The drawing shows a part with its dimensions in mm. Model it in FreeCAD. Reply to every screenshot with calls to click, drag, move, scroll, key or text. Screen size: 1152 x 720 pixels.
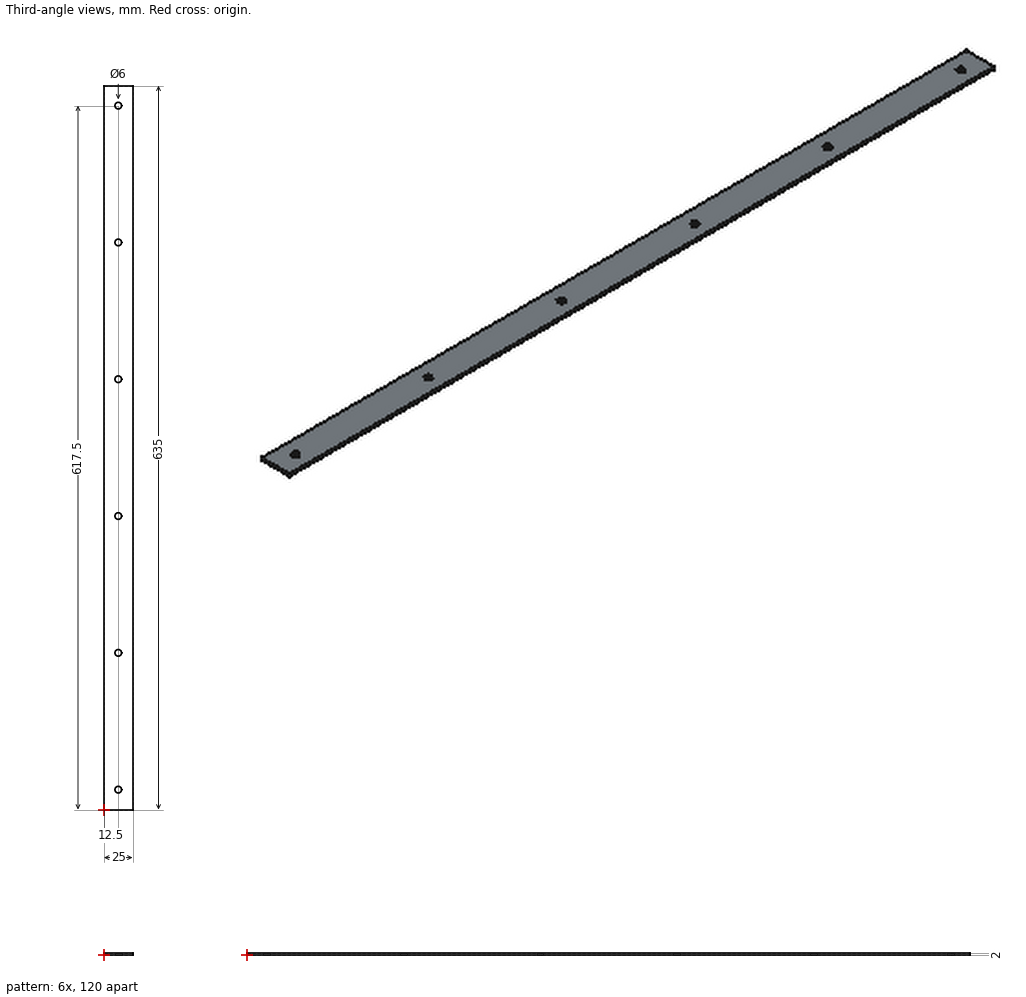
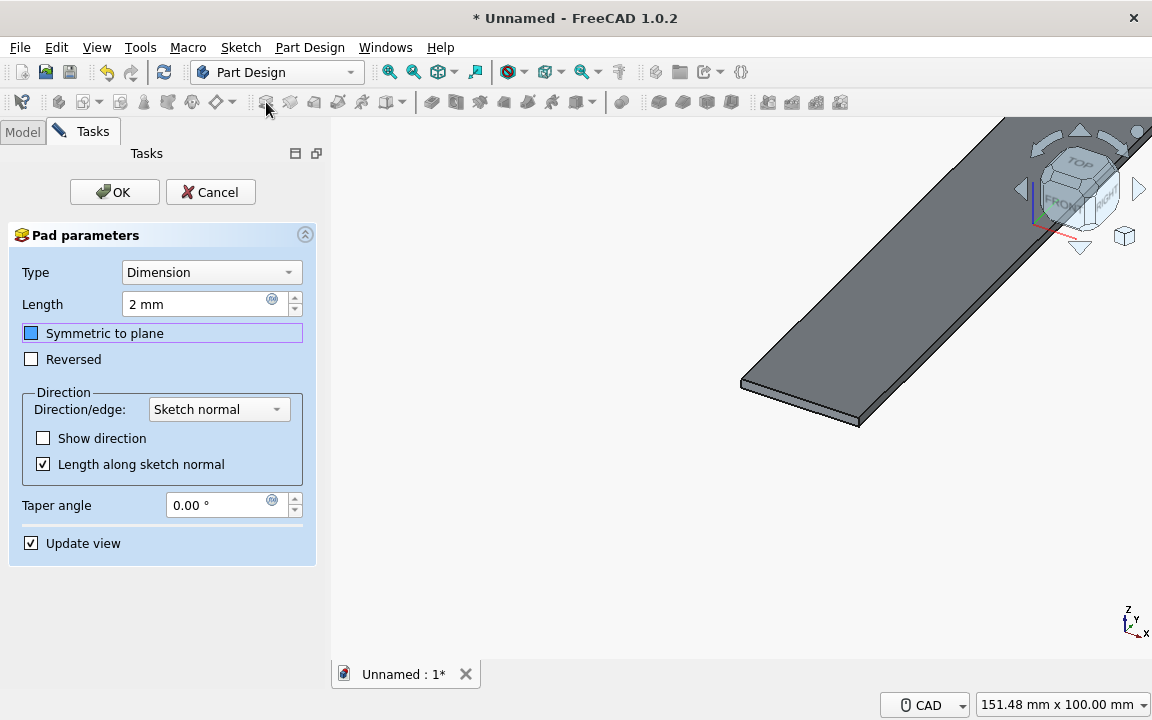
click(115, 192)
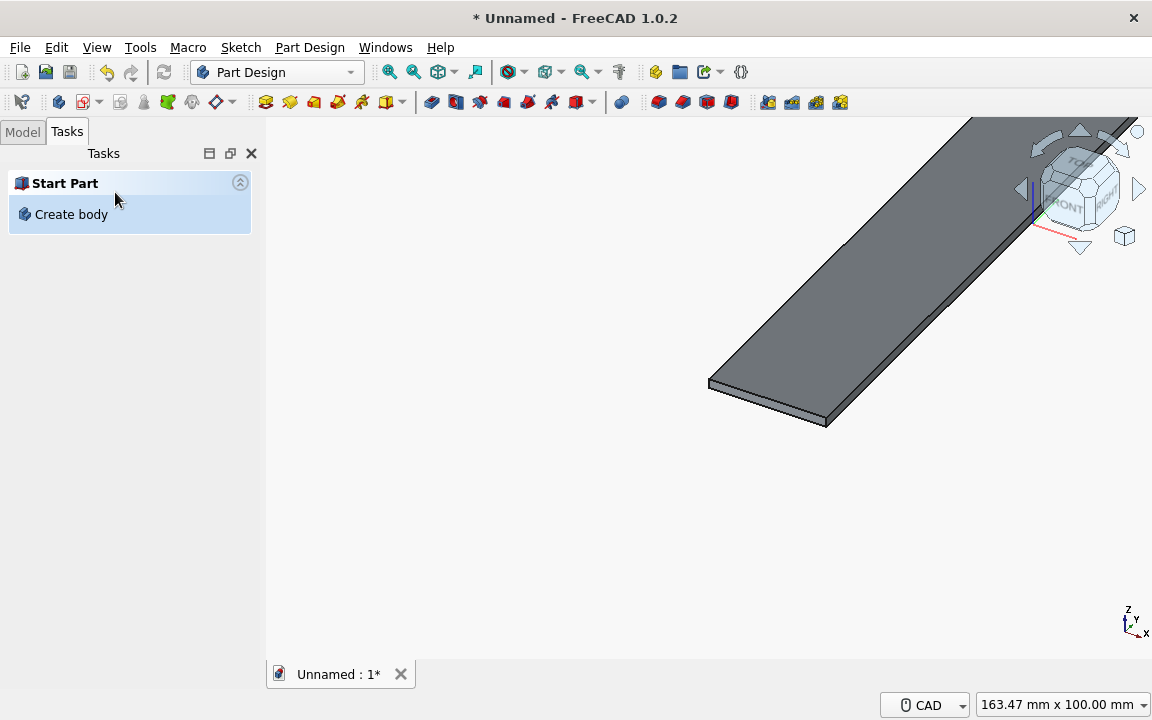
click(390, 72)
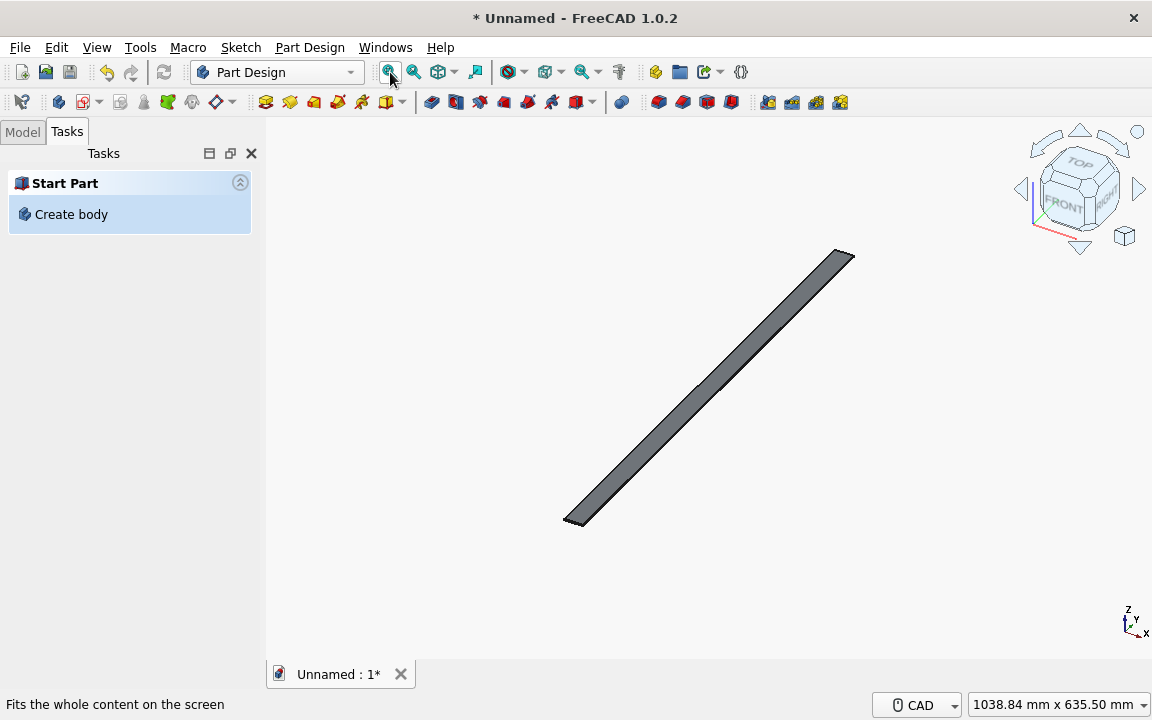
click(786, 309)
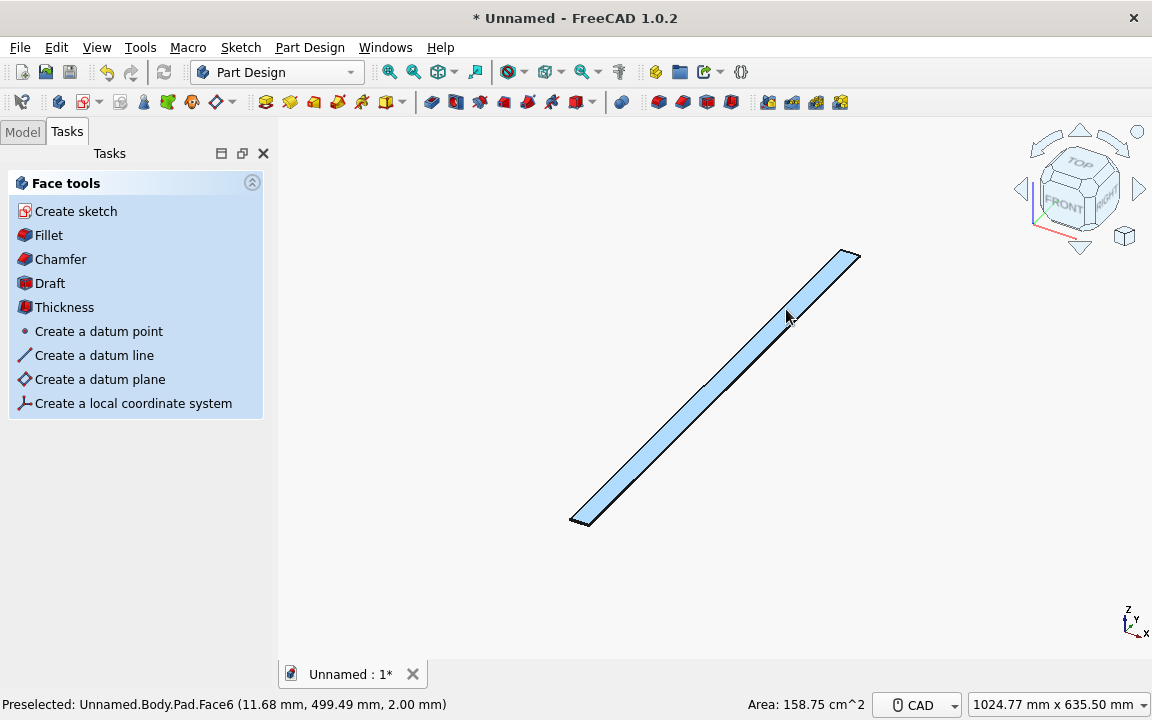
click(84, 102)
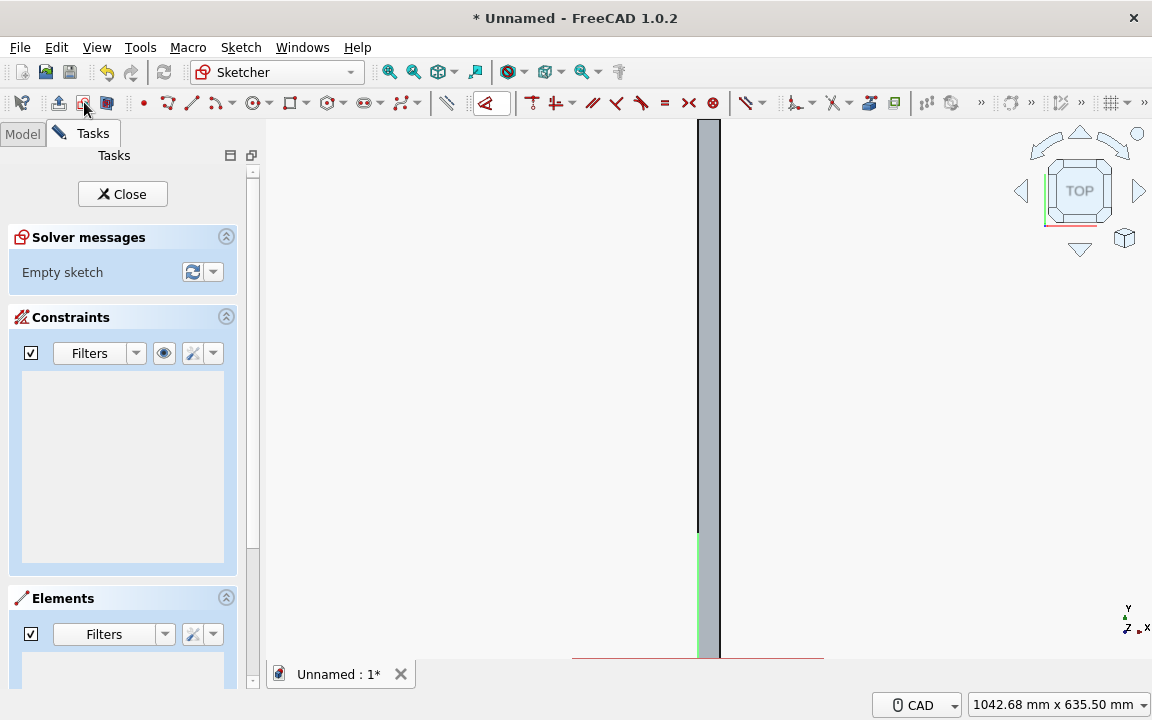
scroll(640, 389, down, 5)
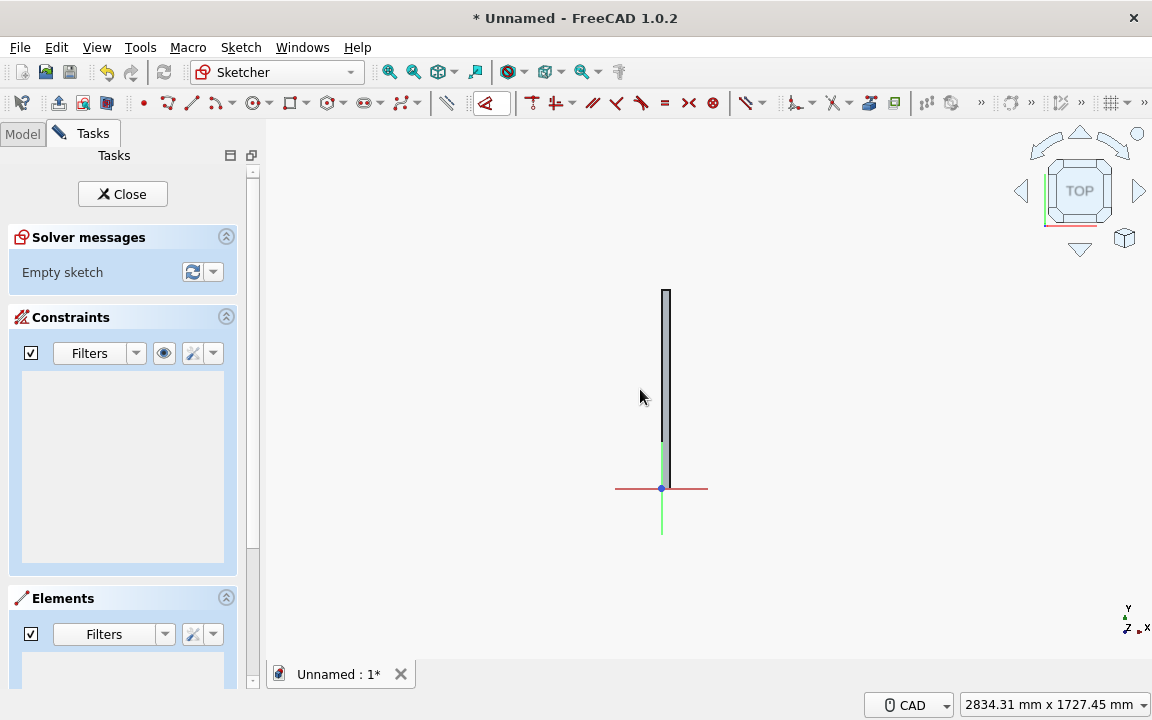
scroll(667, 291, up, 15)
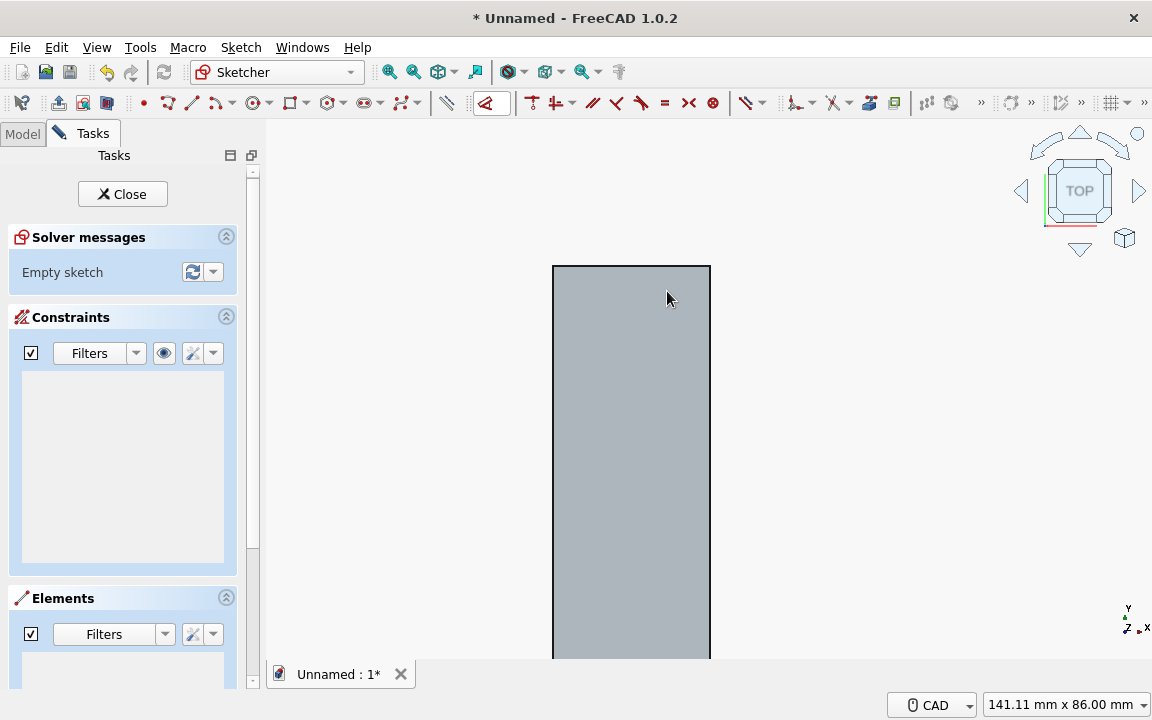
scroll(630, 374, up, 11)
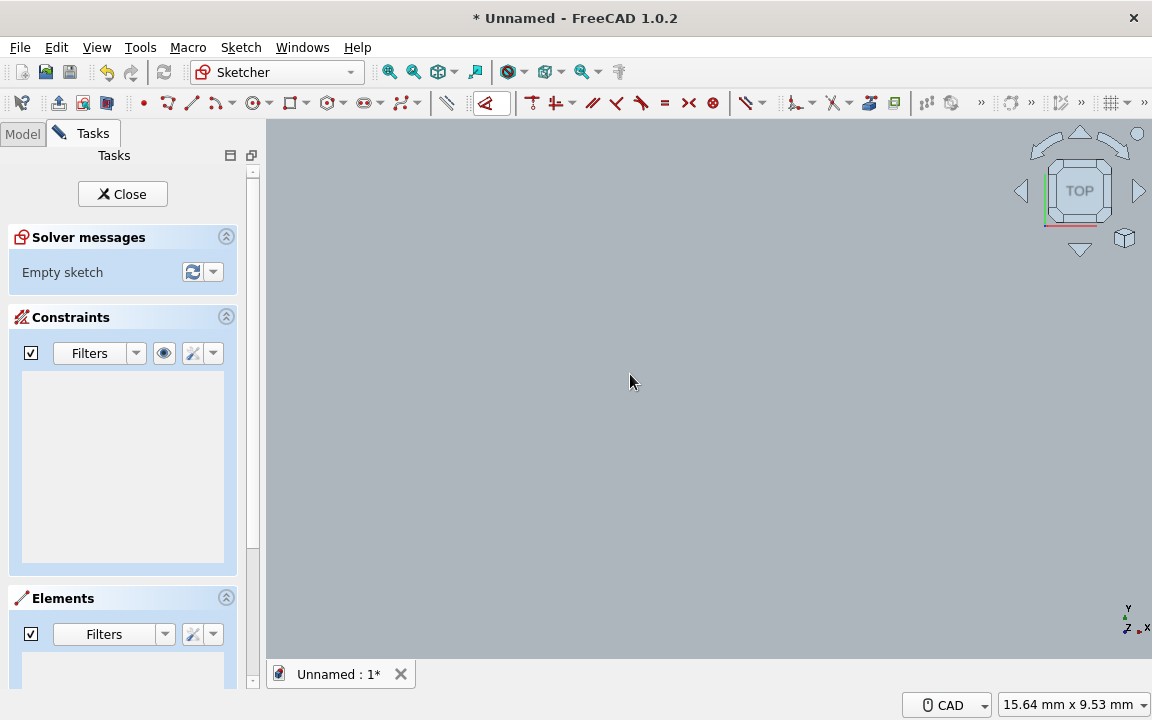
click(254, 104)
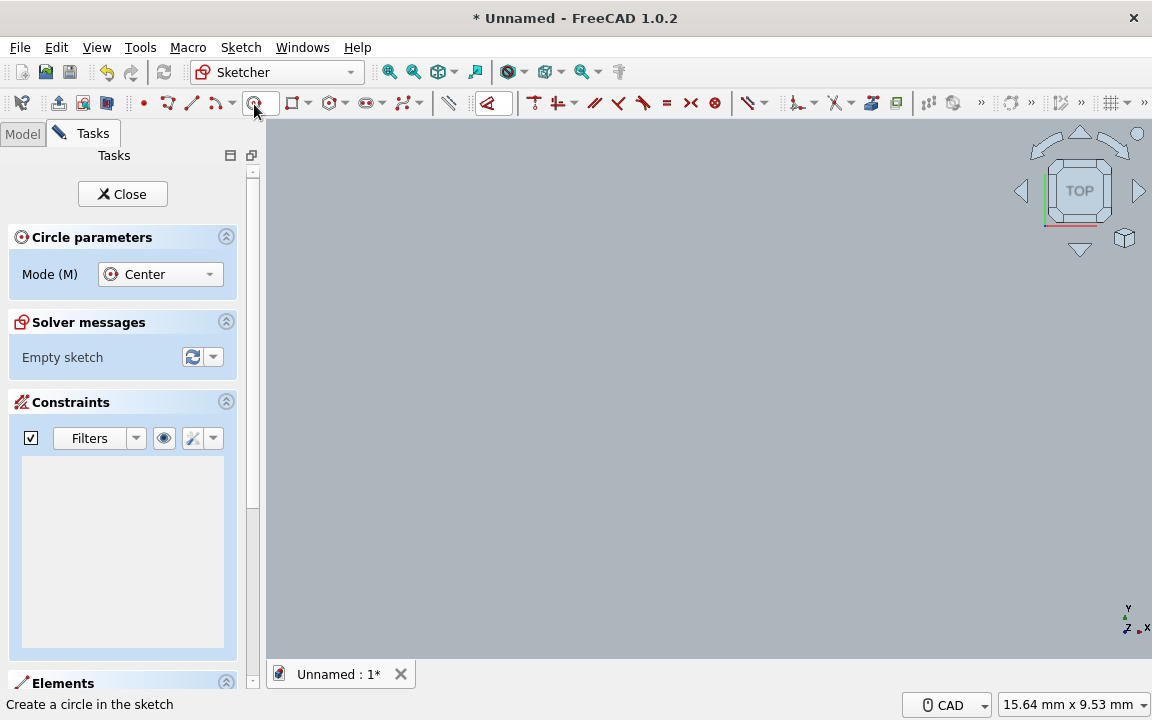
click(638, 389)
click(758, 268)
key(Escape)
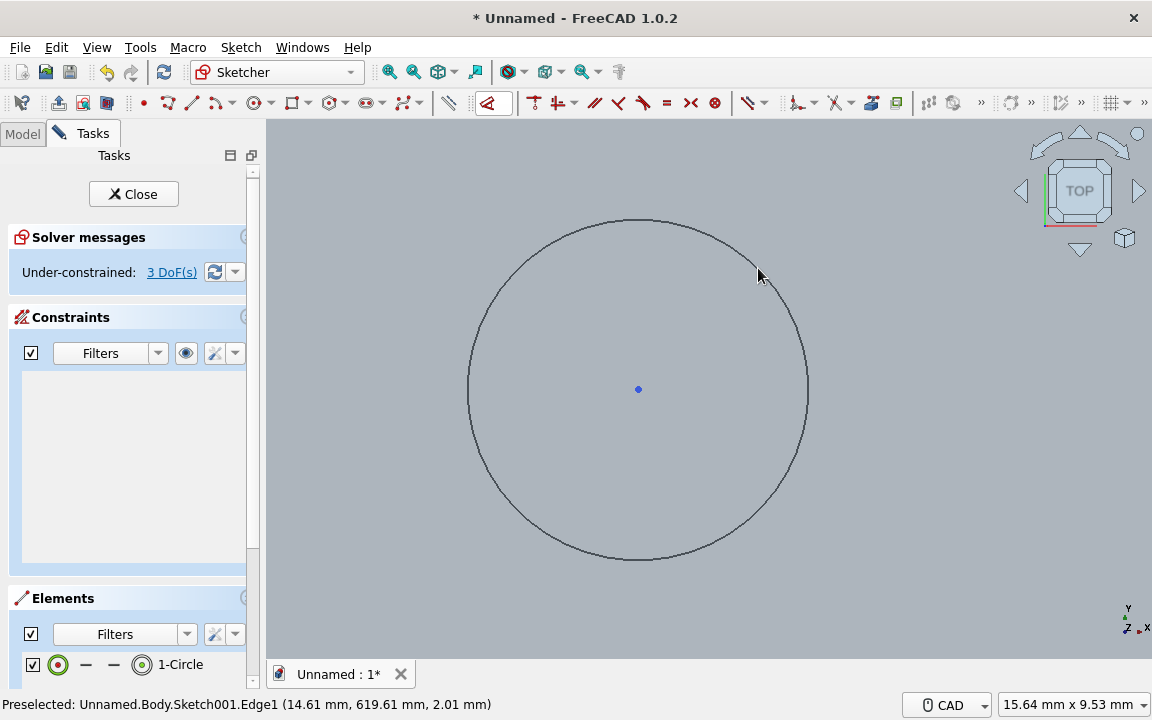
click(758, 269)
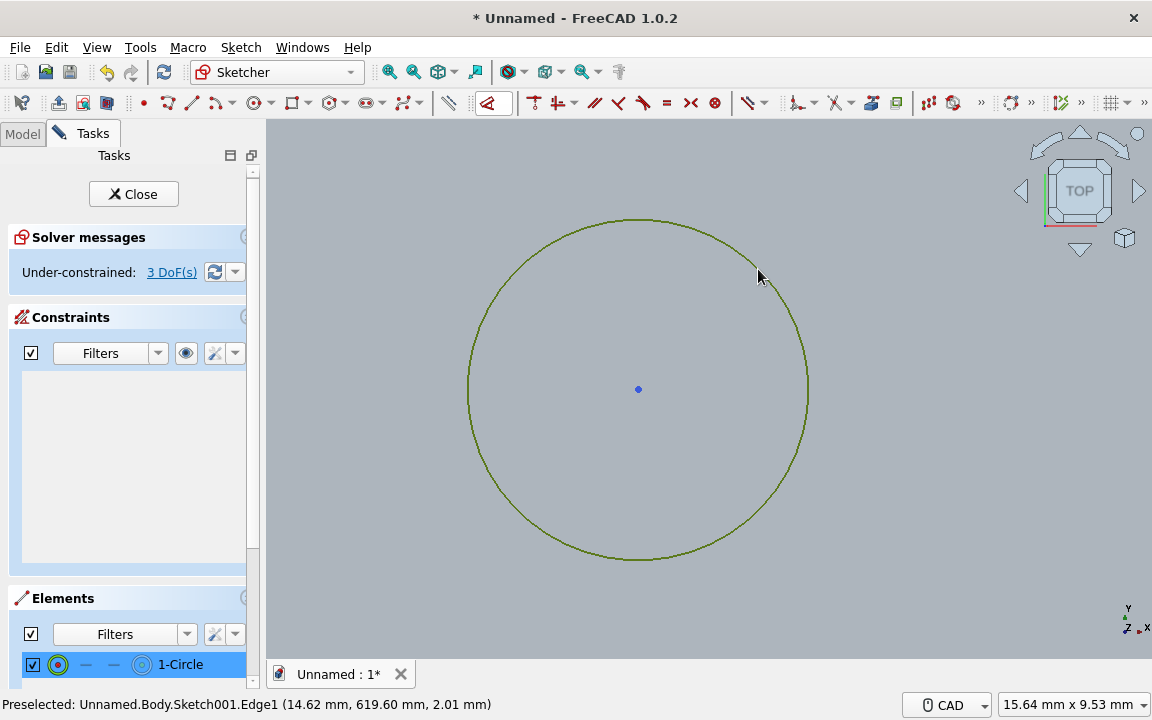
click(506, 104)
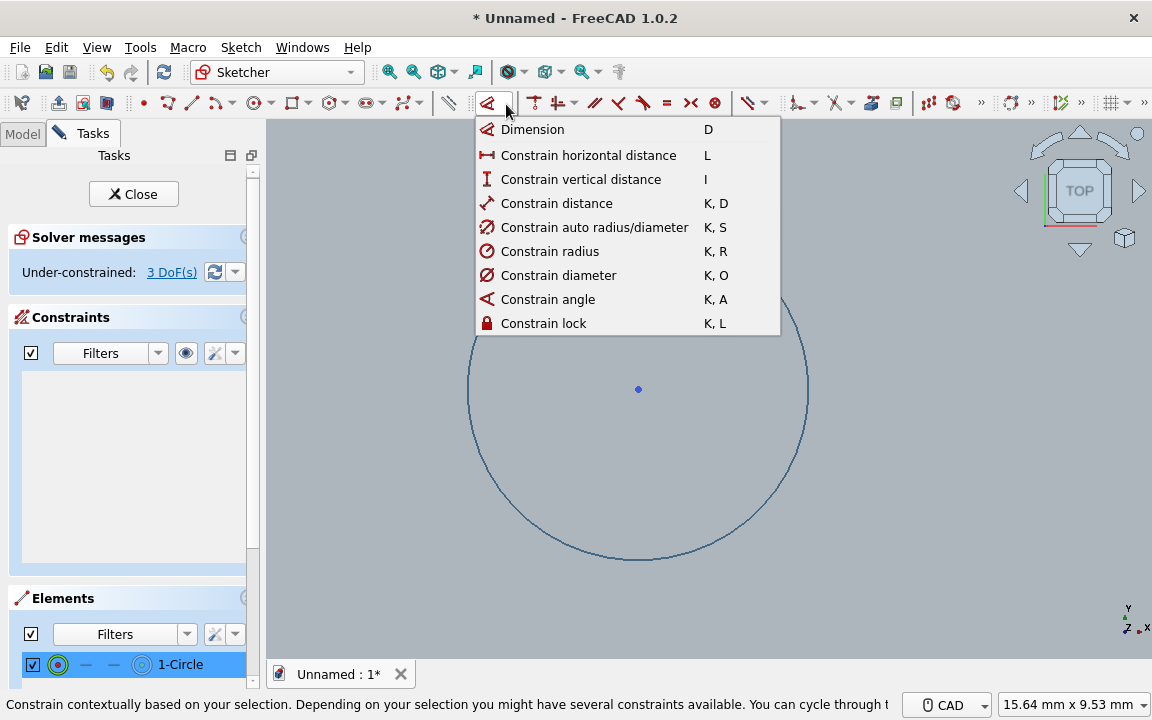
click(628, 275)